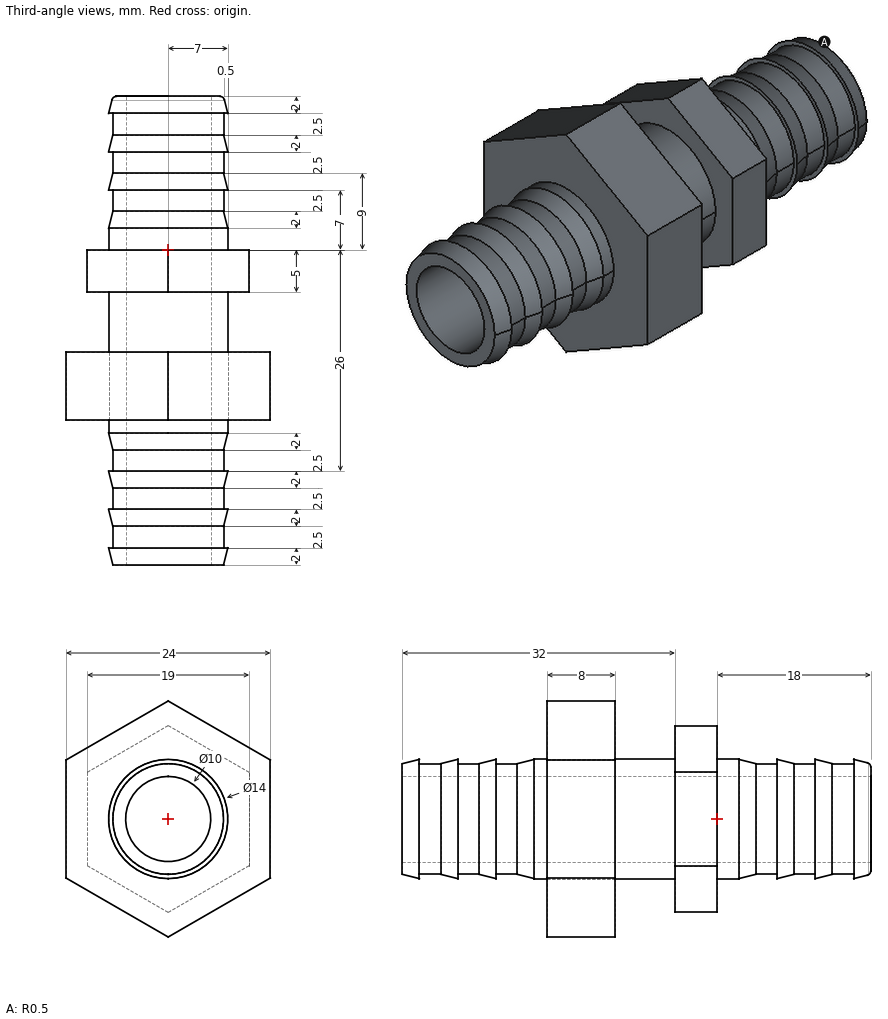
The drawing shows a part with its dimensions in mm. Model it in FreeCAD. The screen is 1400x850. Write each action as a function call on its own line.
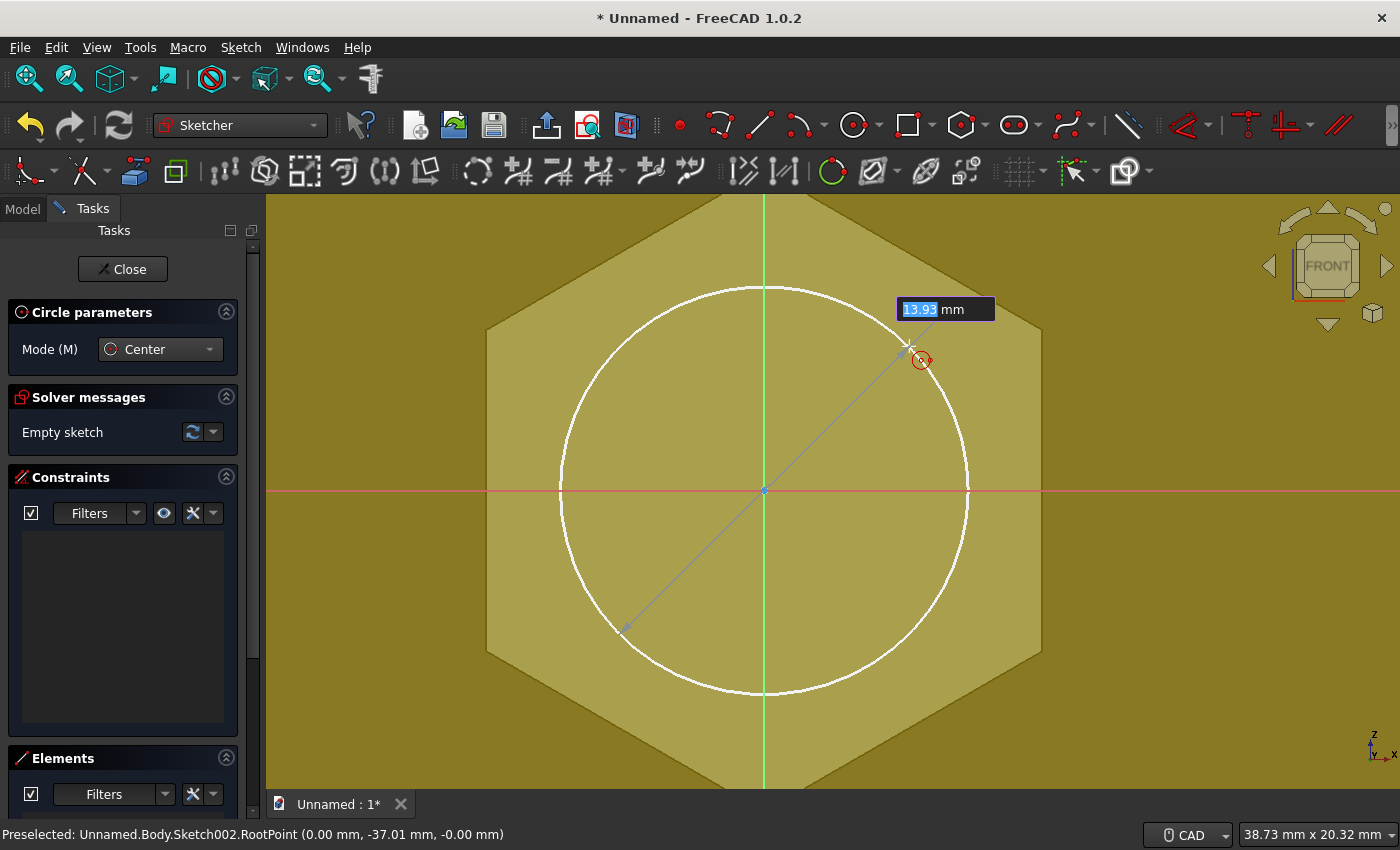
text(14)
key(Return)
key(Escape)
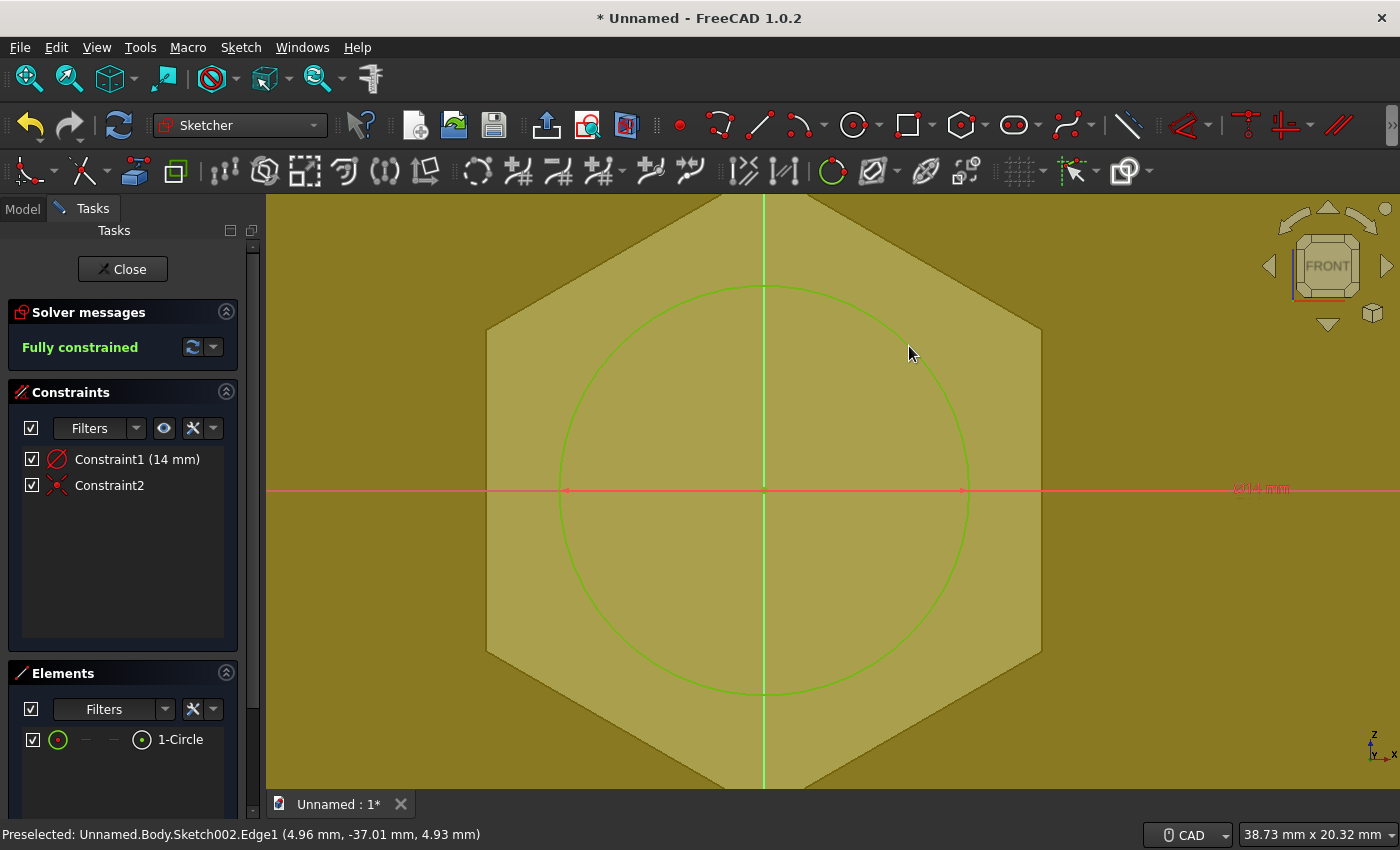
click(123, 269)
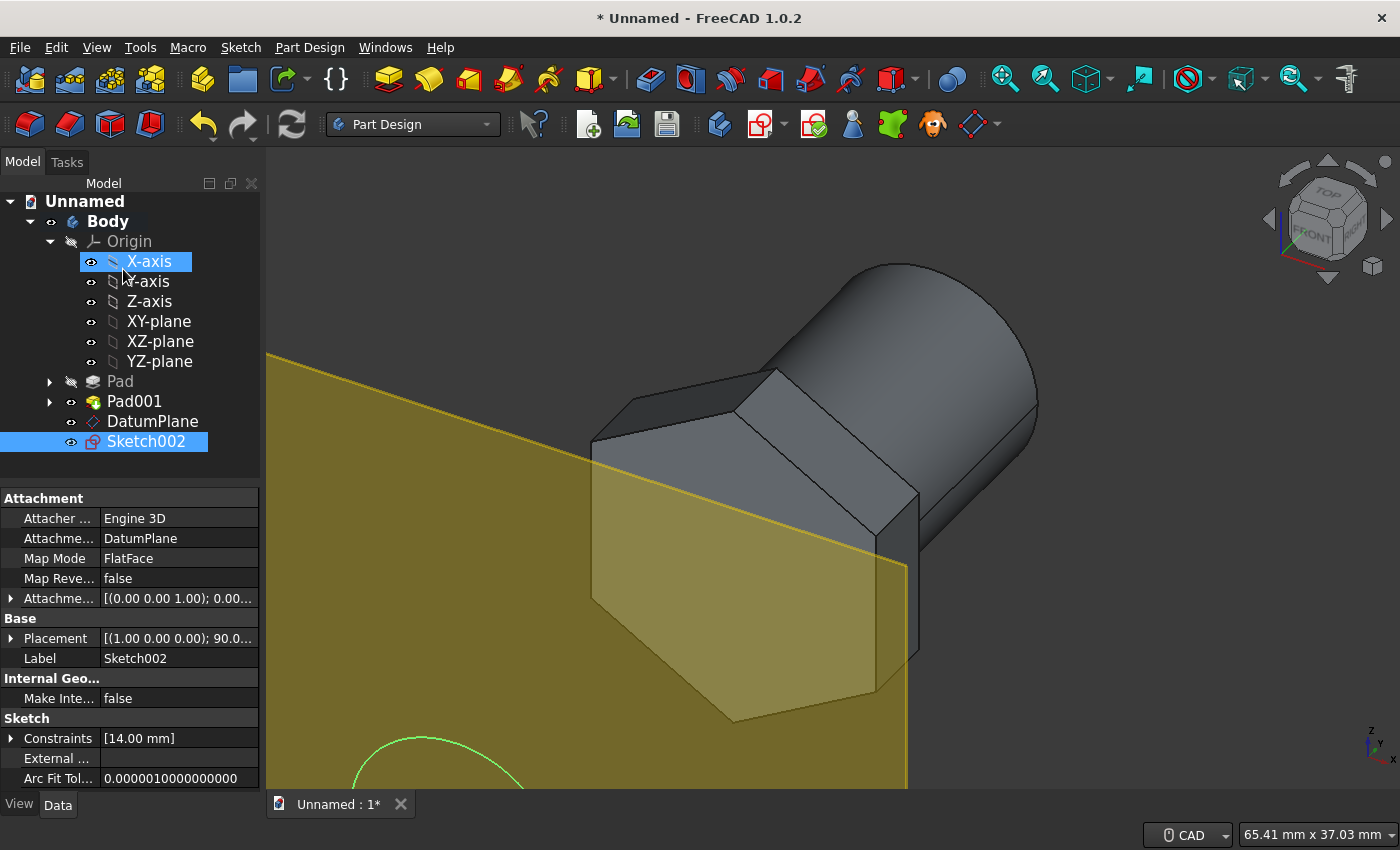
click(390, 80)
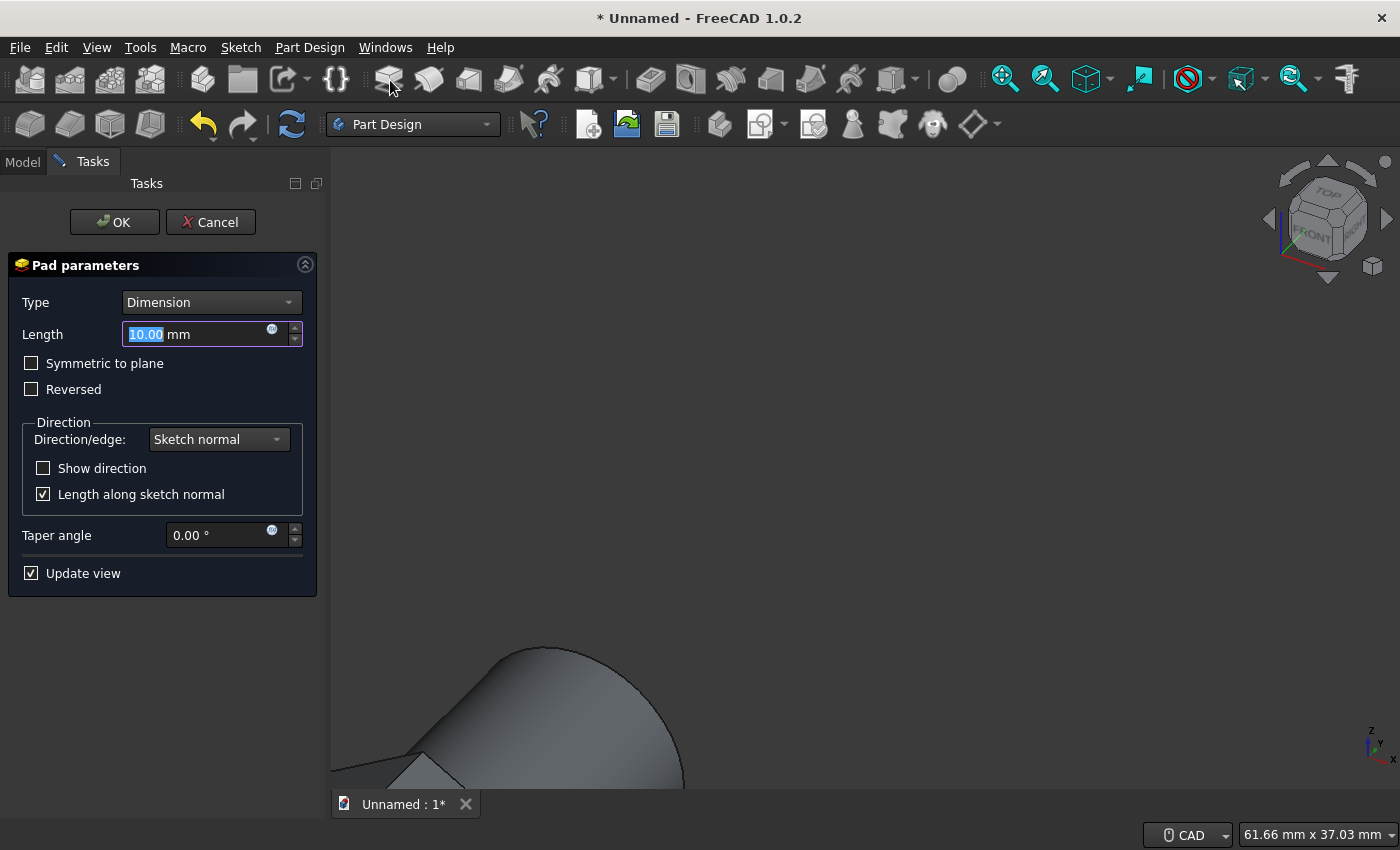
text(32)
key(Tab)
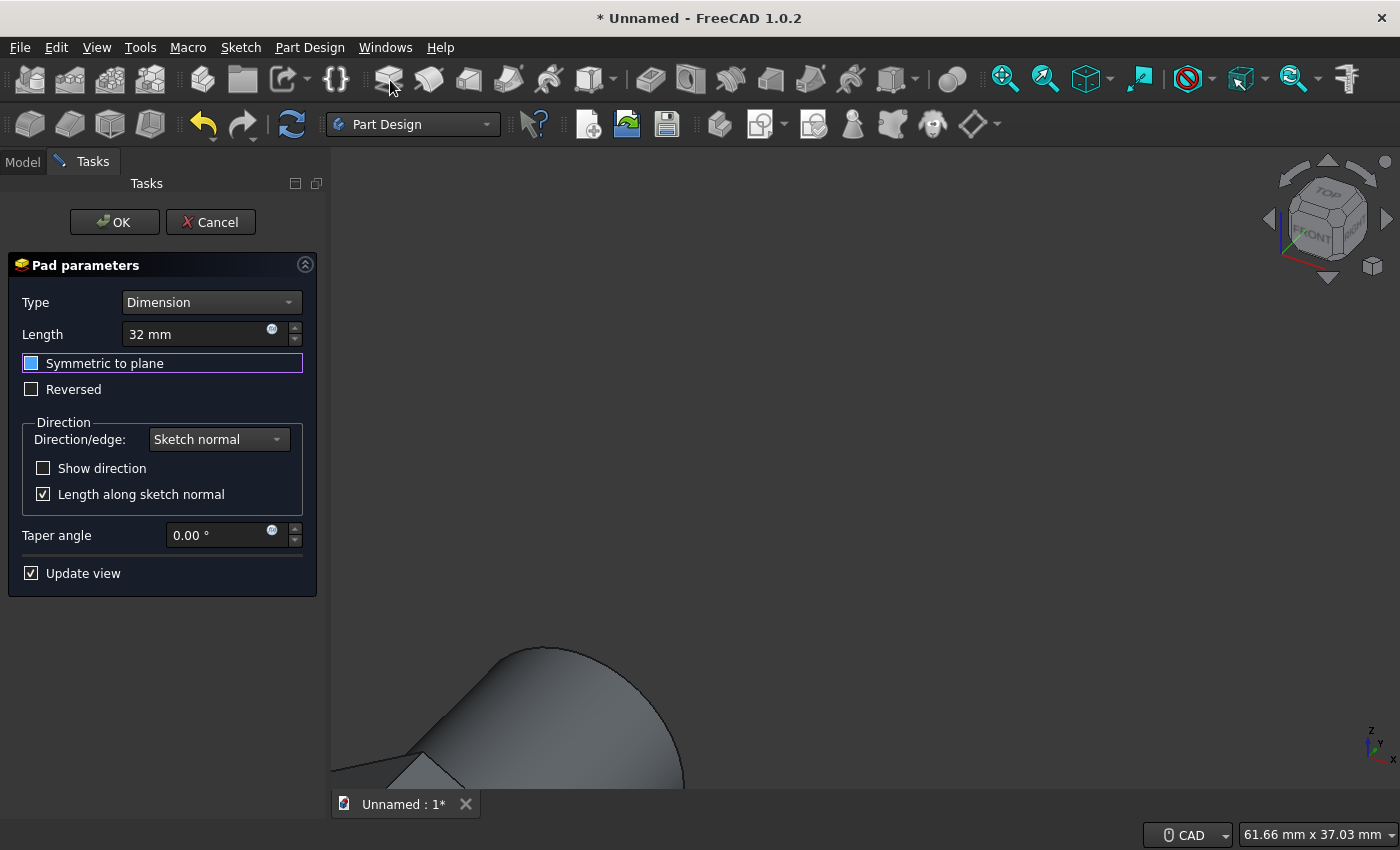
click(30, 389)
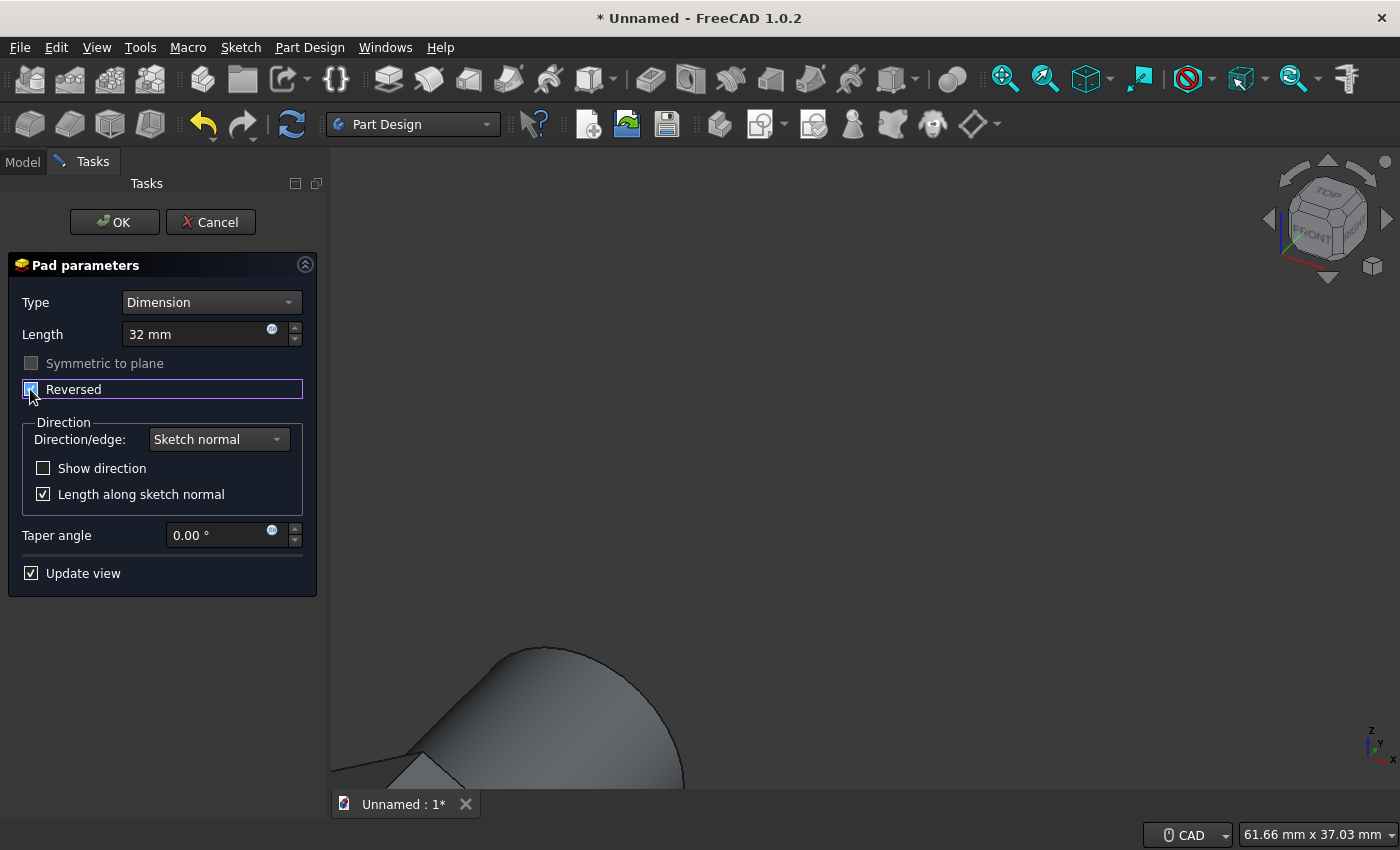
click(115, 222)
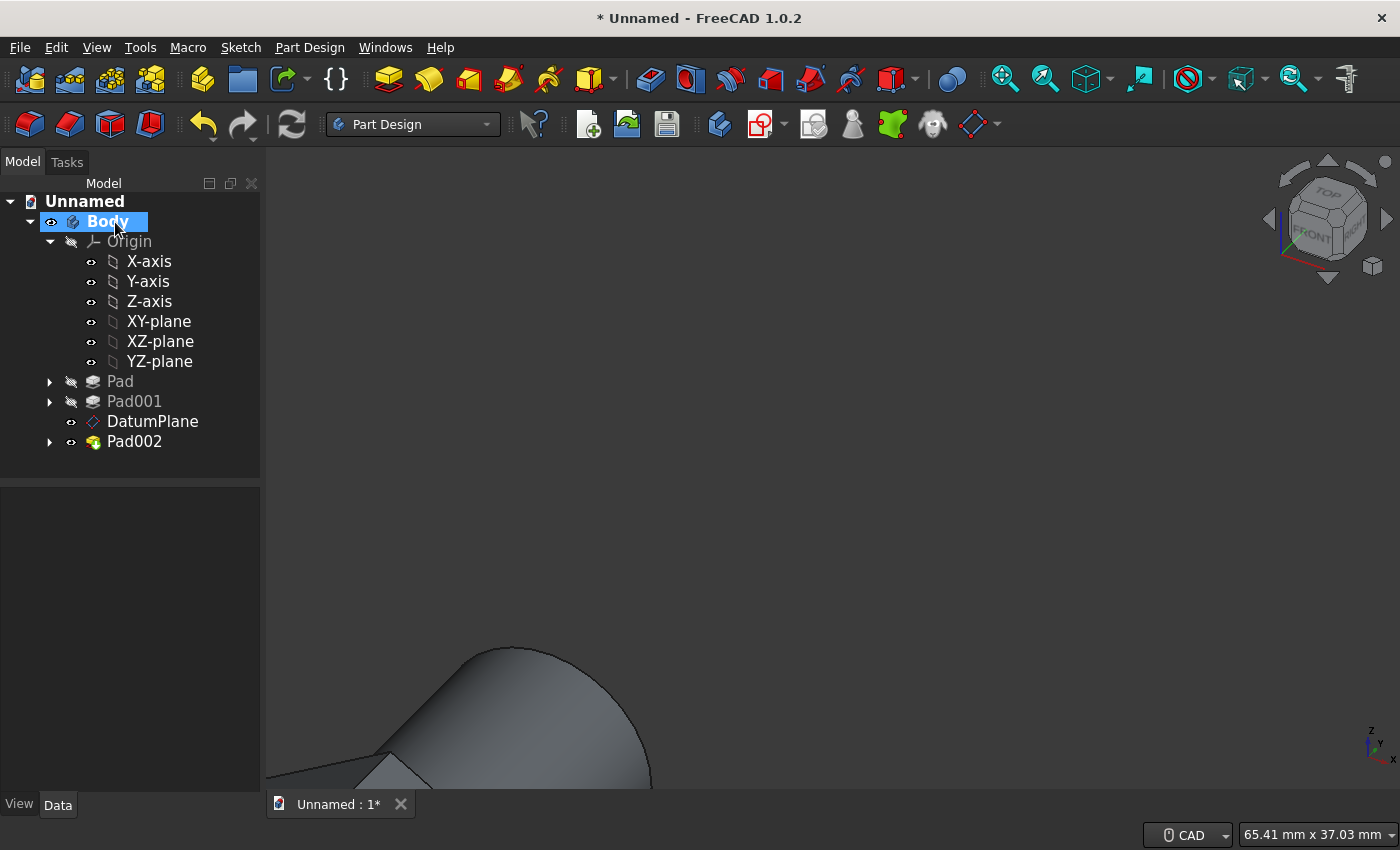
click(116, 422)
key(space)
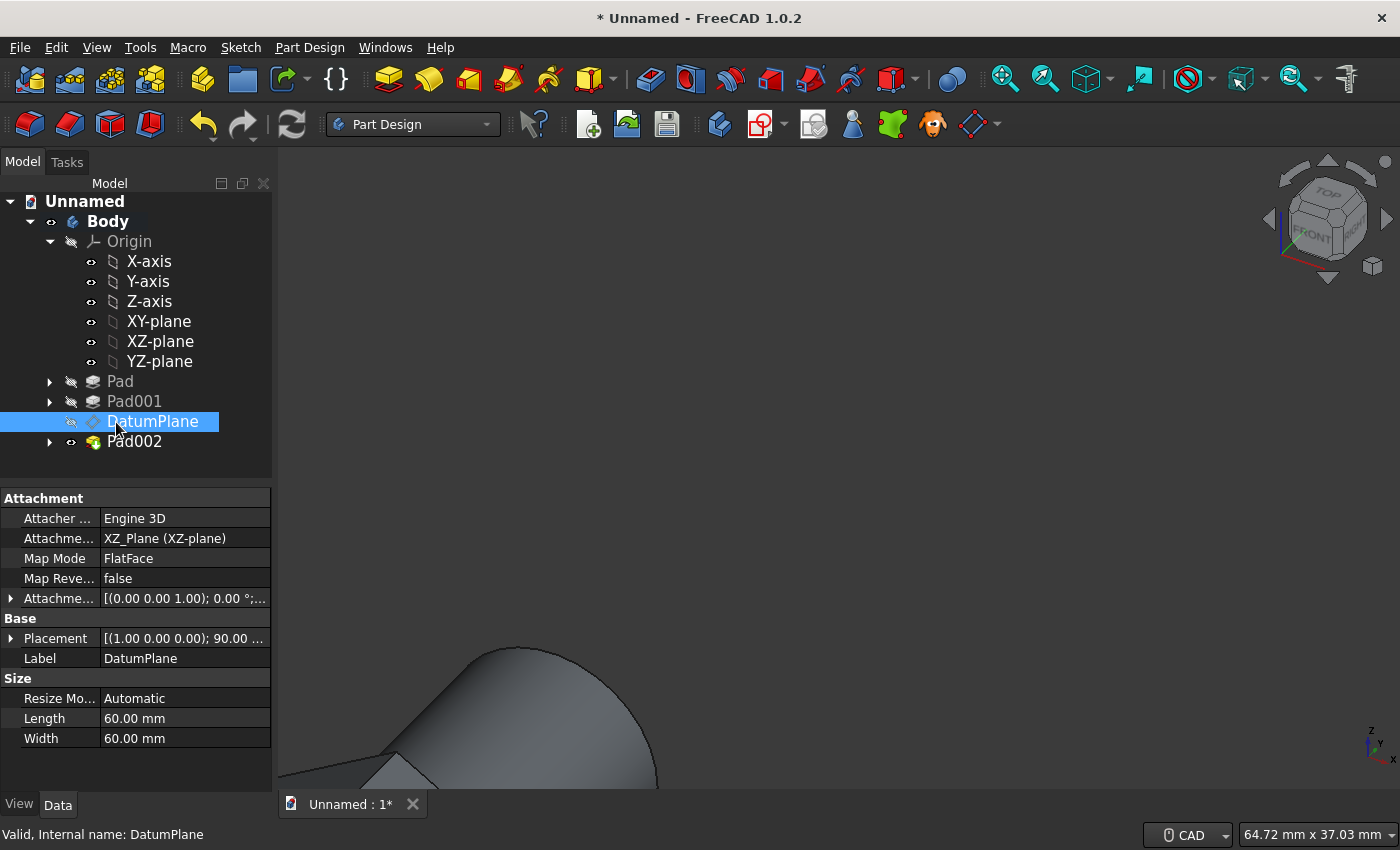
click(1006, 80)